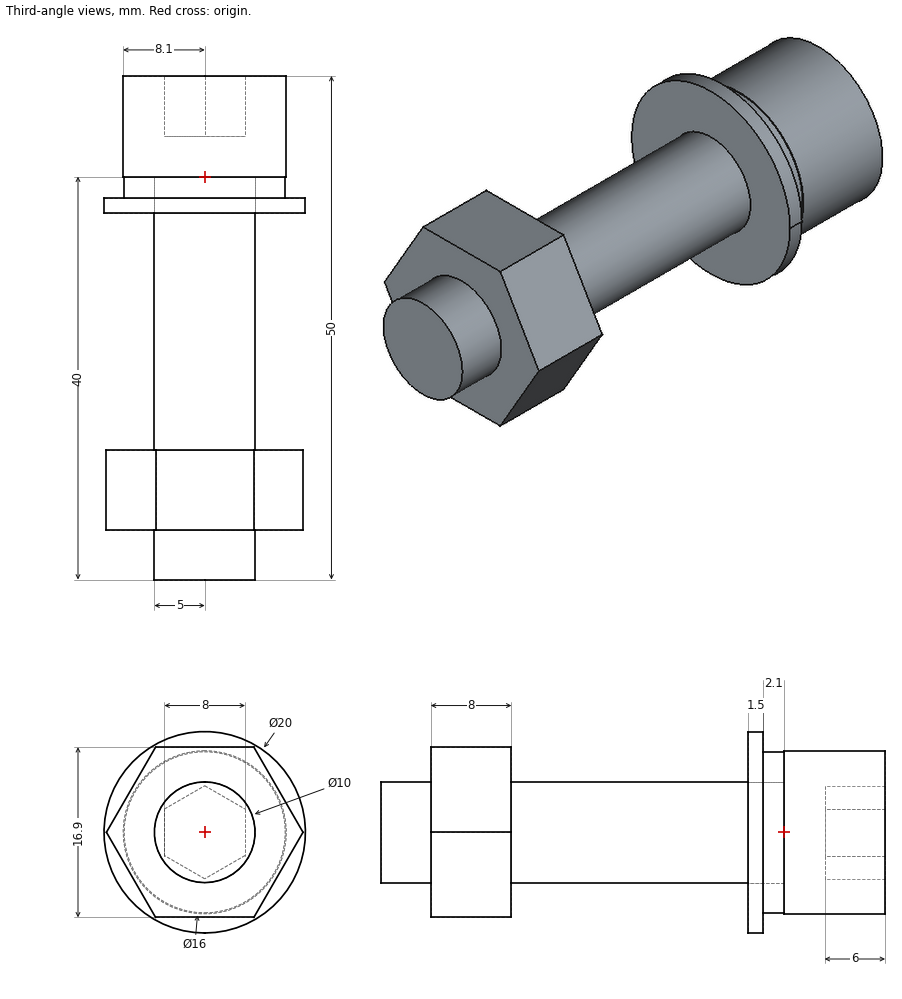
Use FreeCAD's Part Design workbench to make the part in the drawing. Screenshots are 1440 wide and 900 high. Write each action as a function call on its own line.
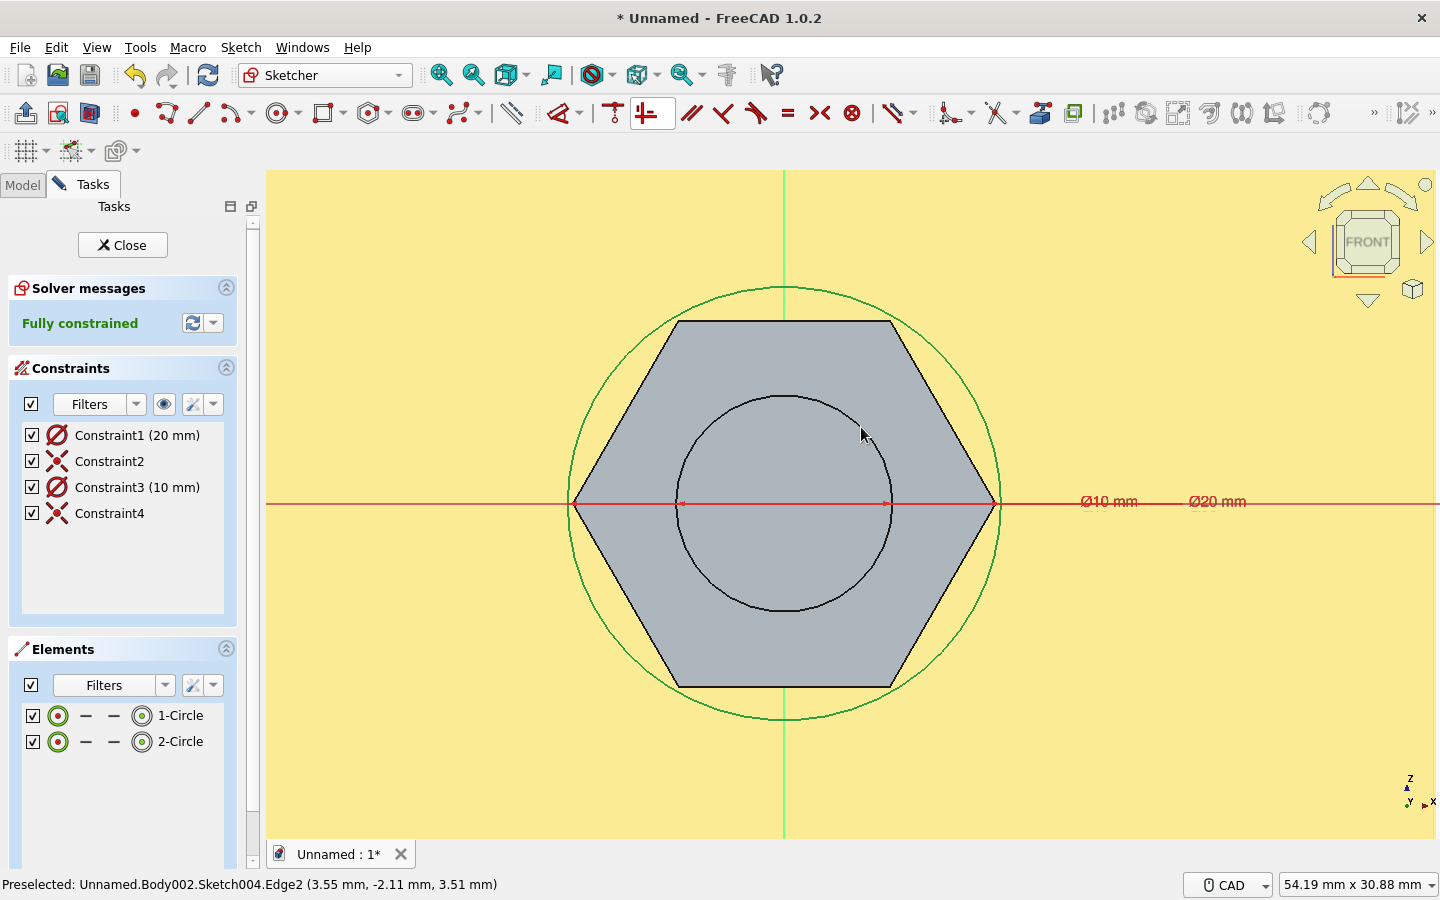
click(123, 245)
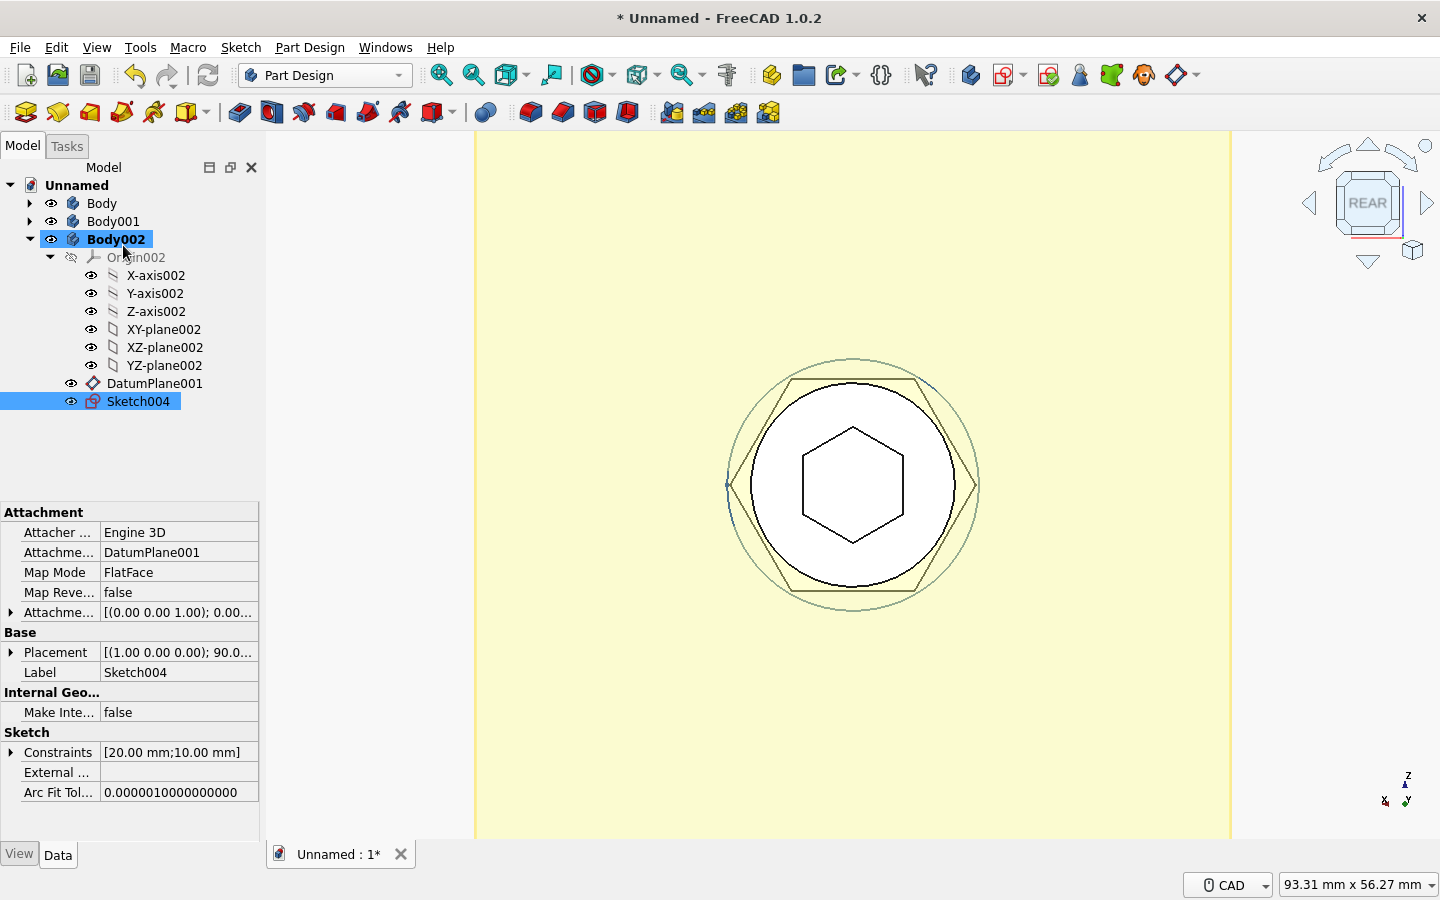
click(26, 112)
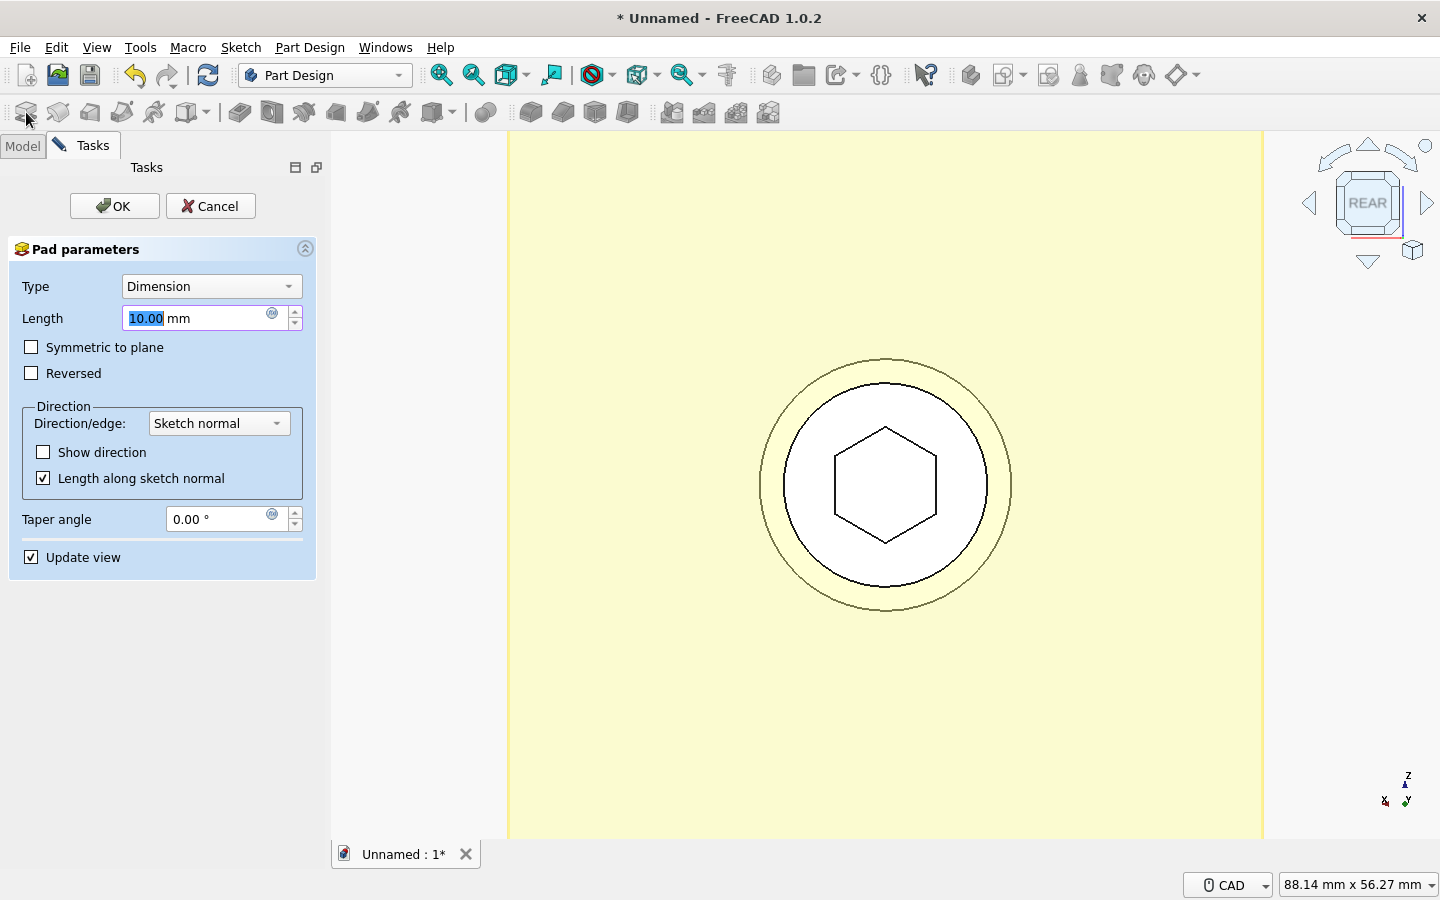
text(1.5)
key(Tab)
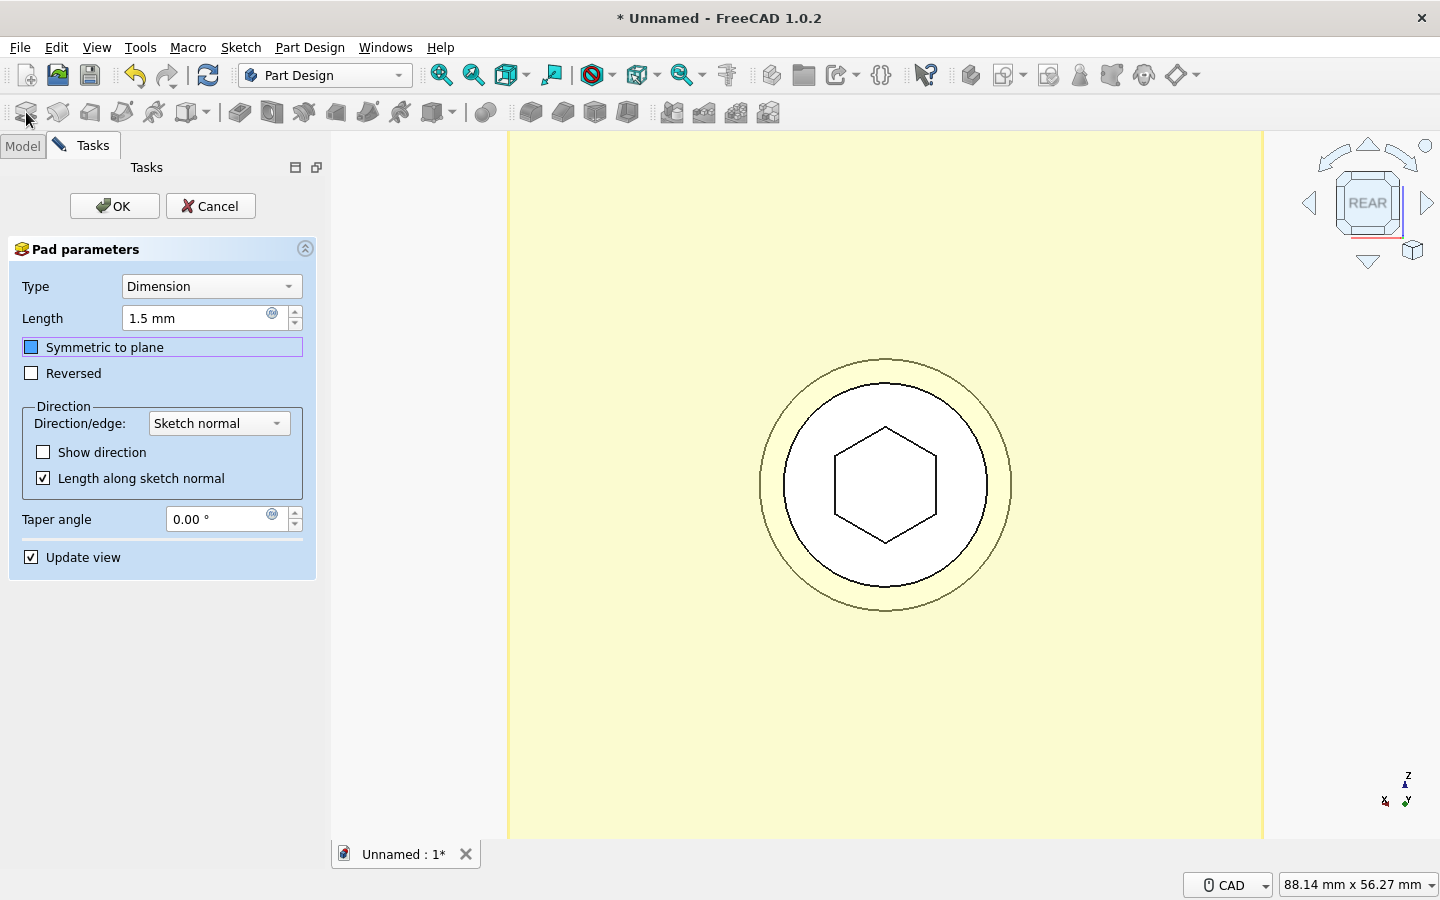
click(115, 206)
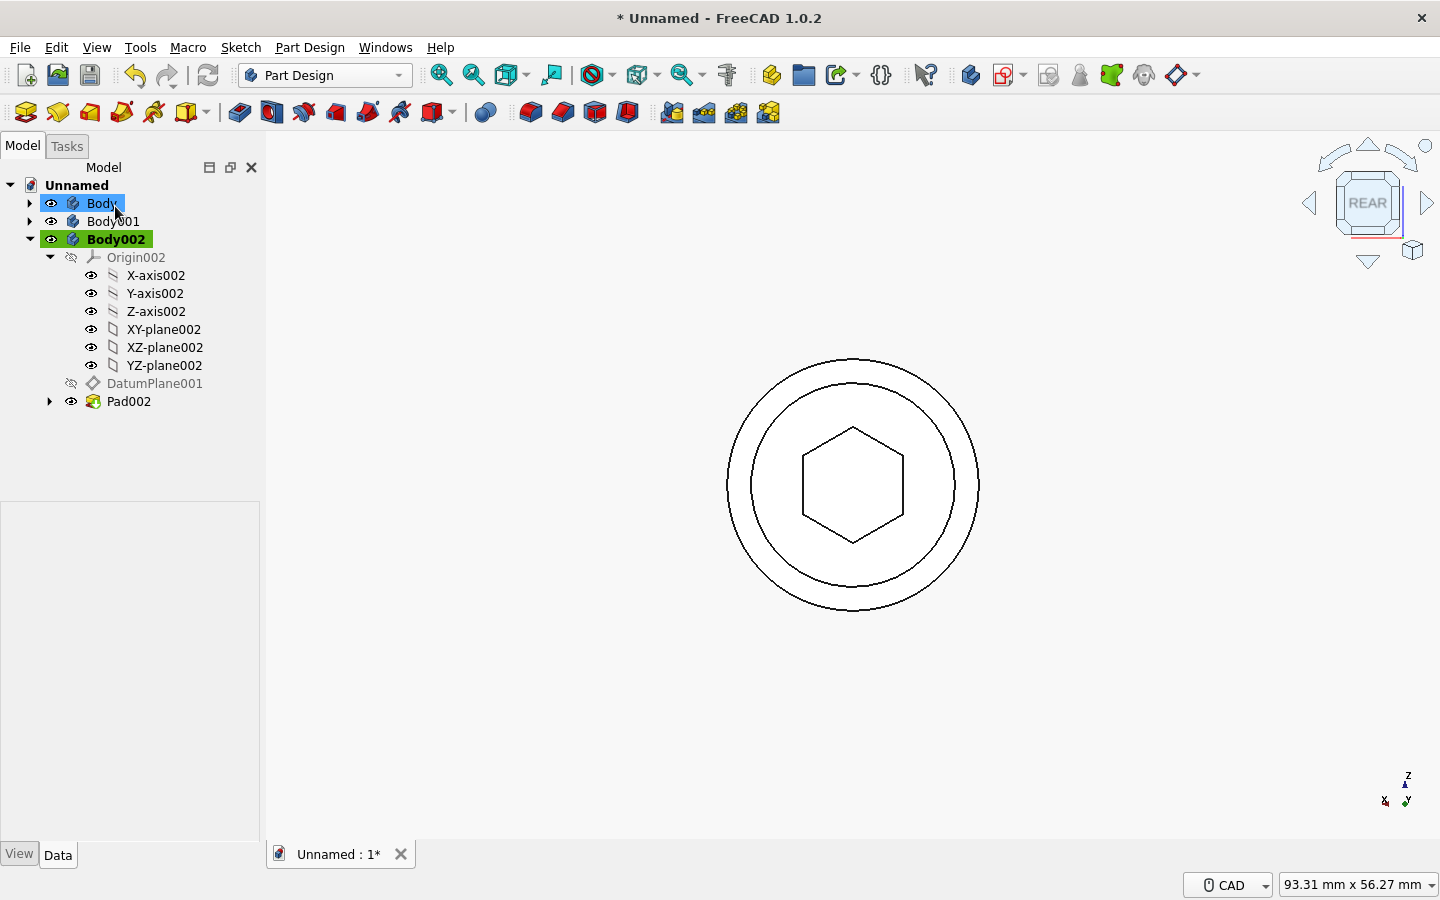
key(0)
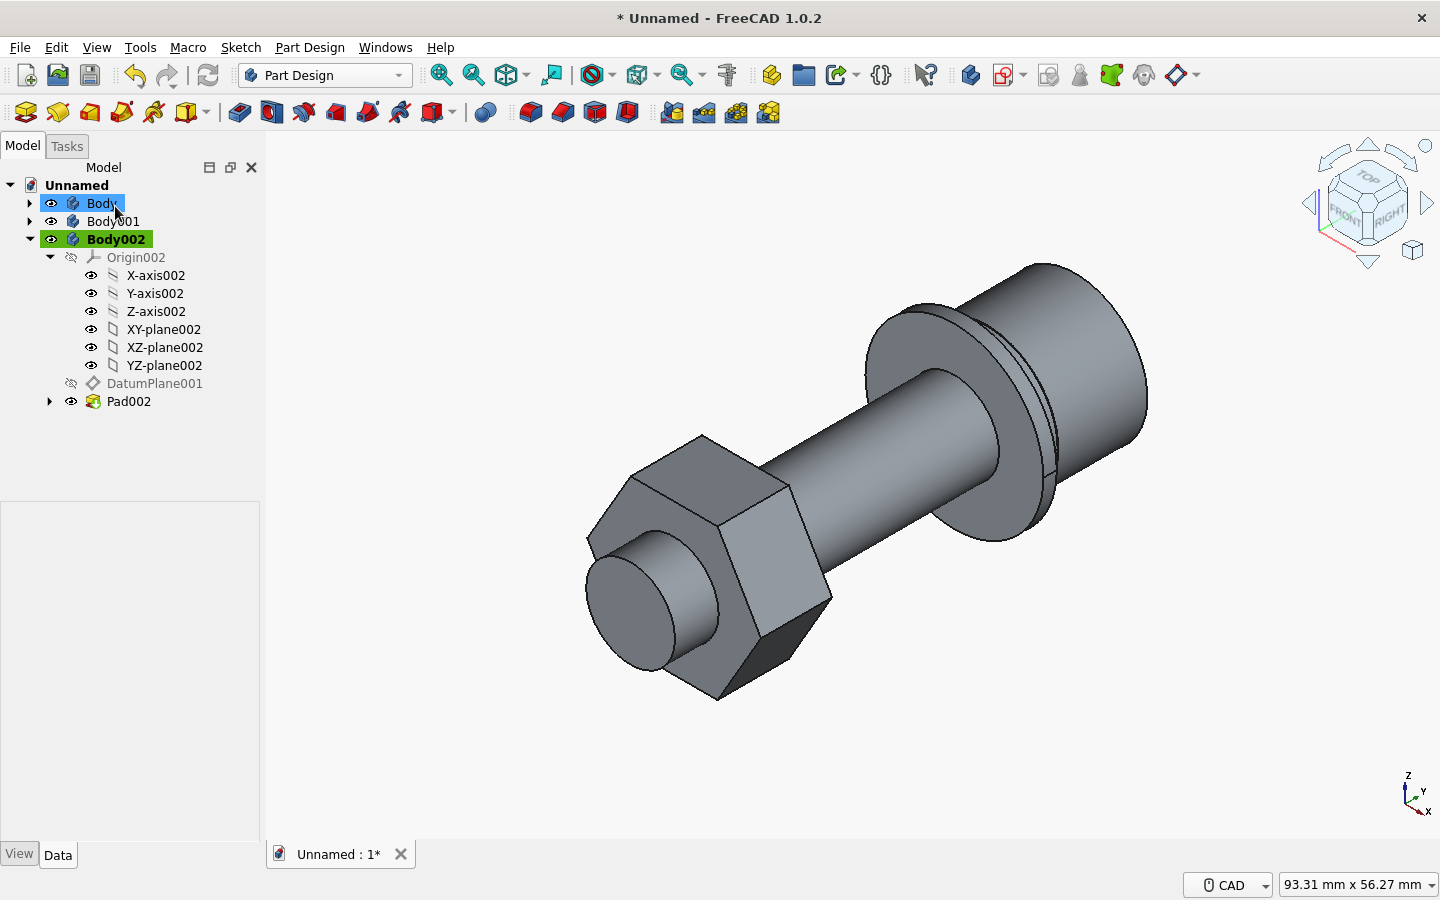
click(442, 76)